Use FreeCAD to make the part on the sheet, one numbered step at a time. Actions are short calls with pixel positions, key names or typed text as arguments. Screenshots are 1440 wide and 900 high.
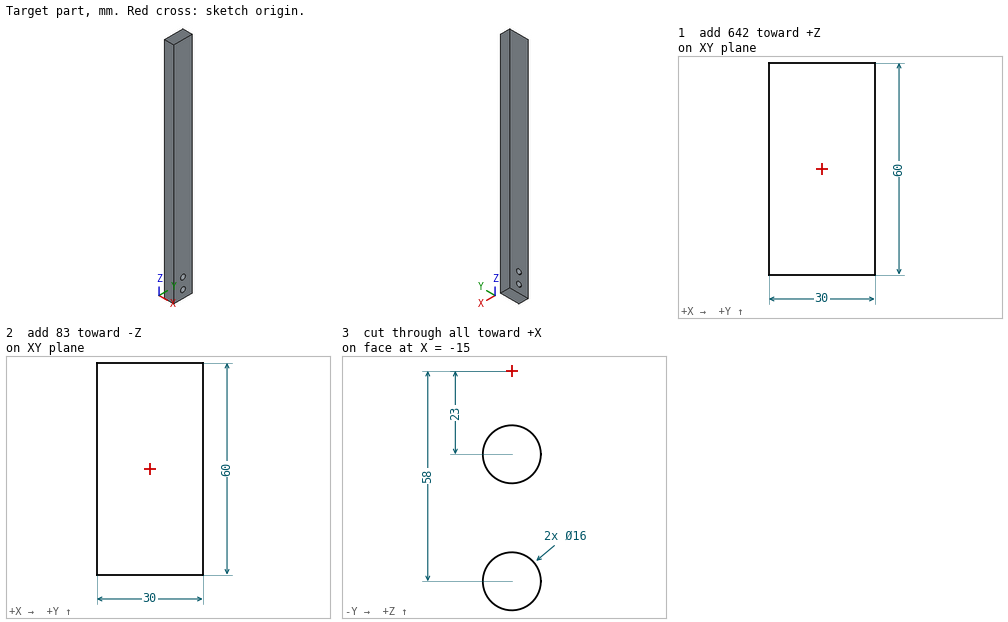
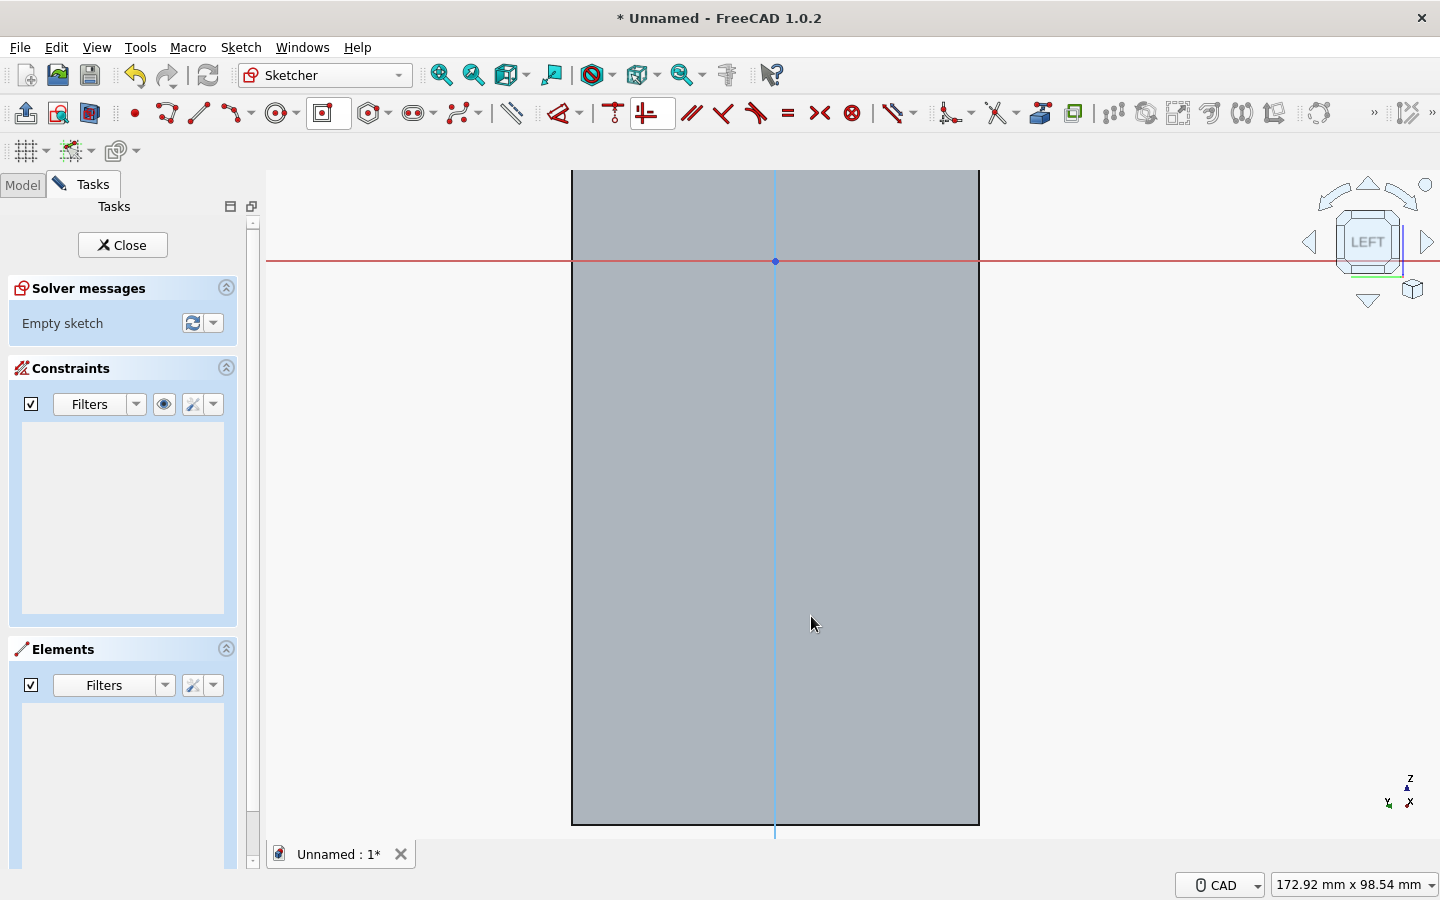
click(276, 114)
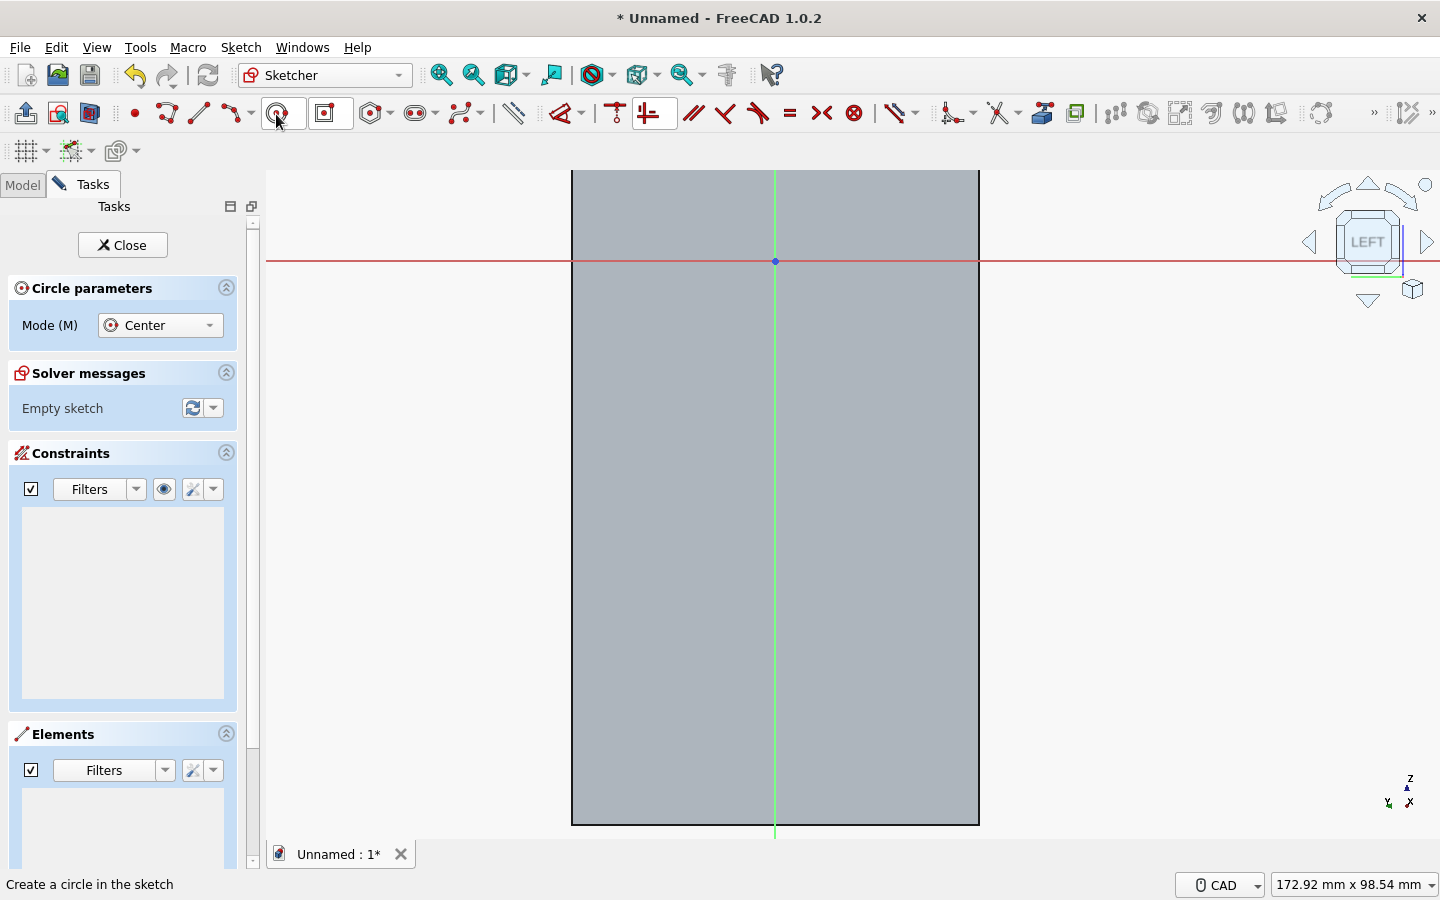
click(775, 655)
move(814, 617)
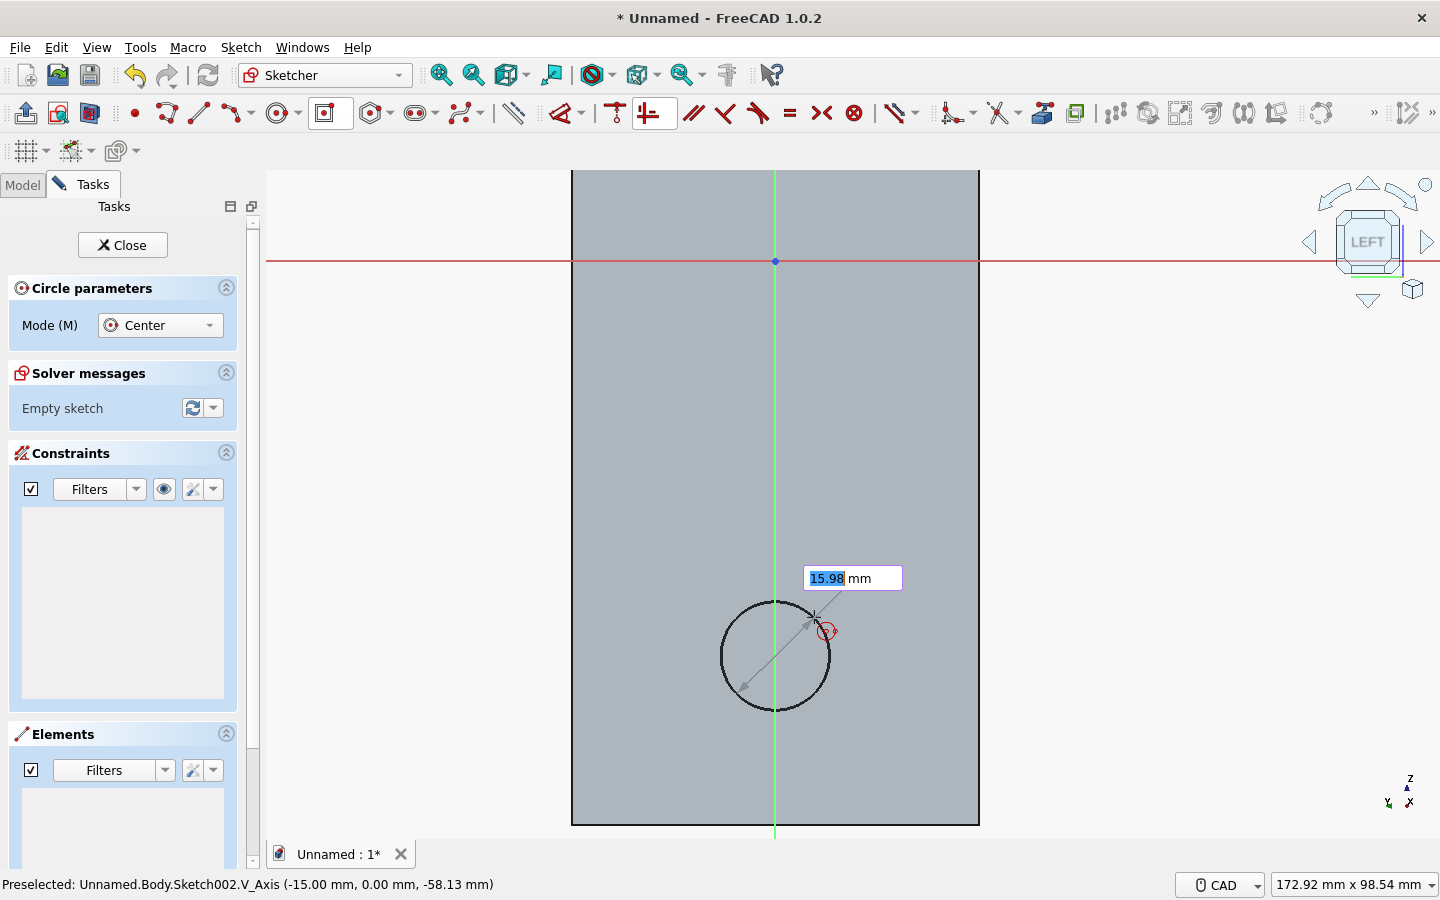
text(16)
key(Return)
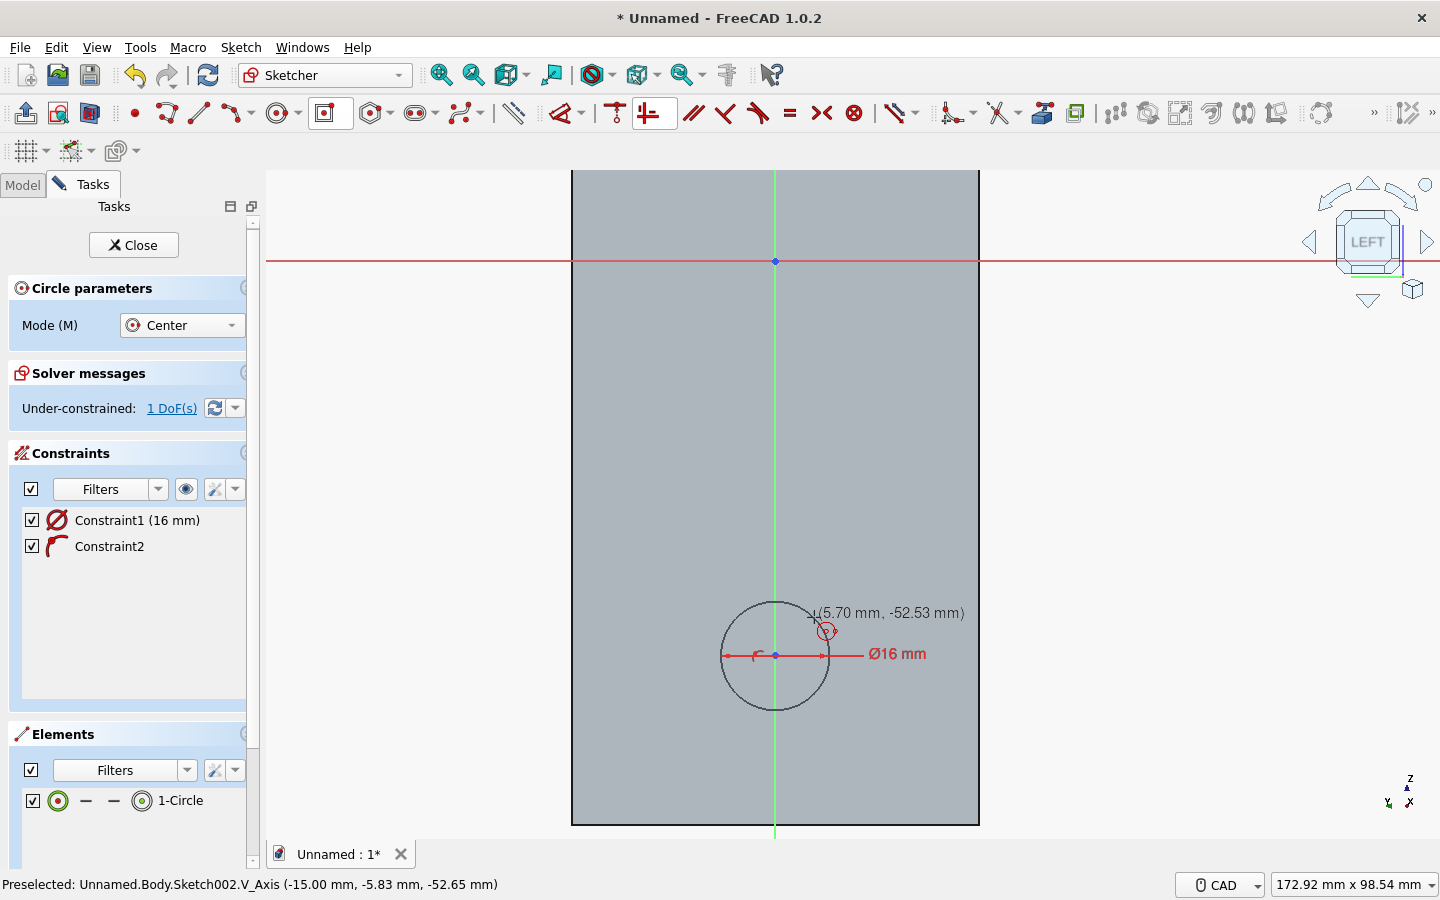
click(775, 417)
move(814, 379)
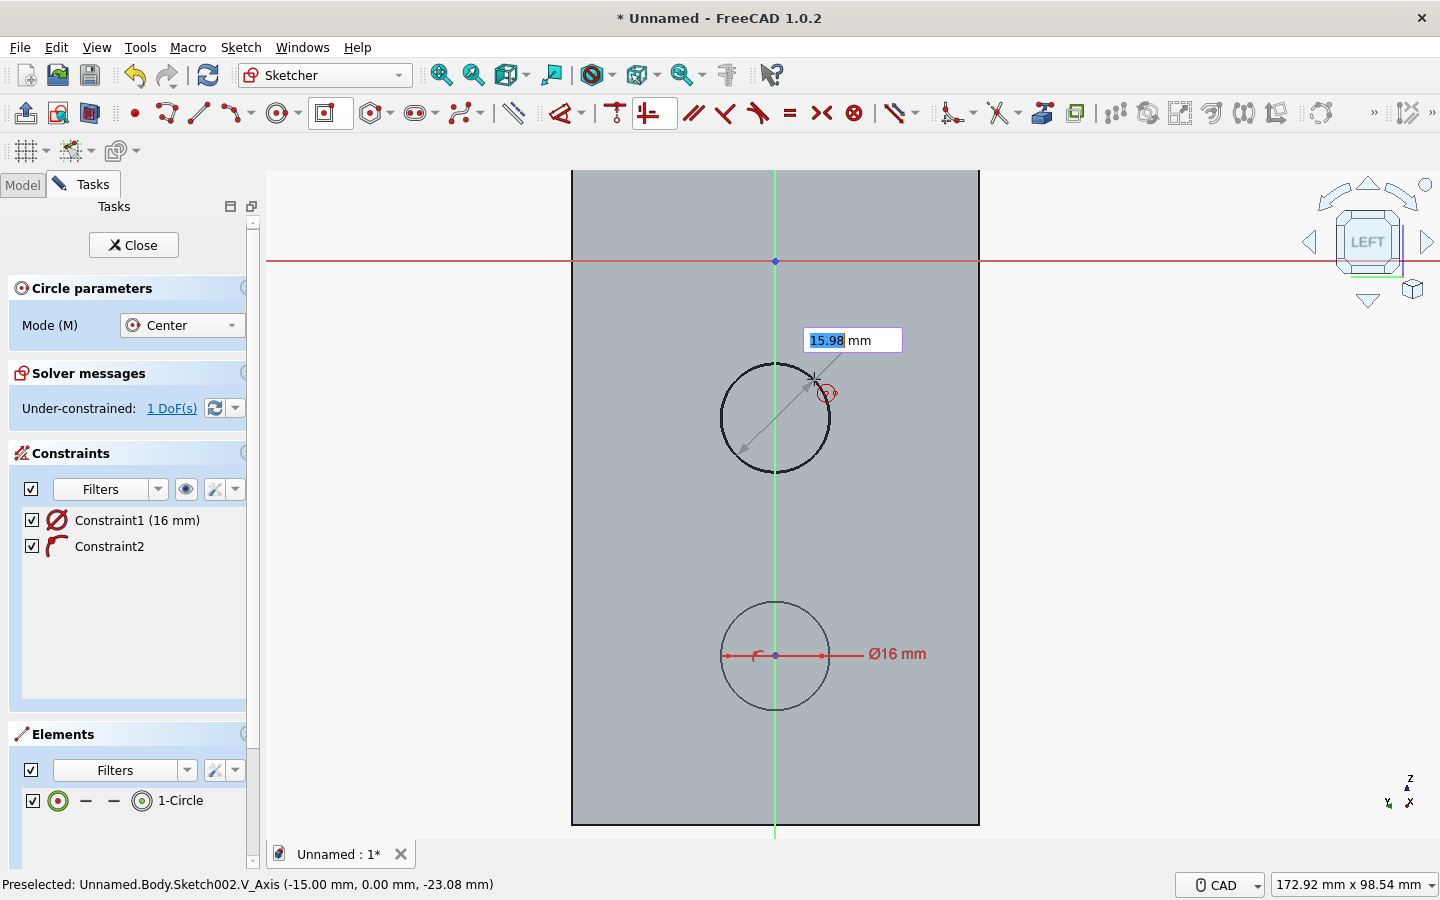
text(16)
key(Return)
key(Escape)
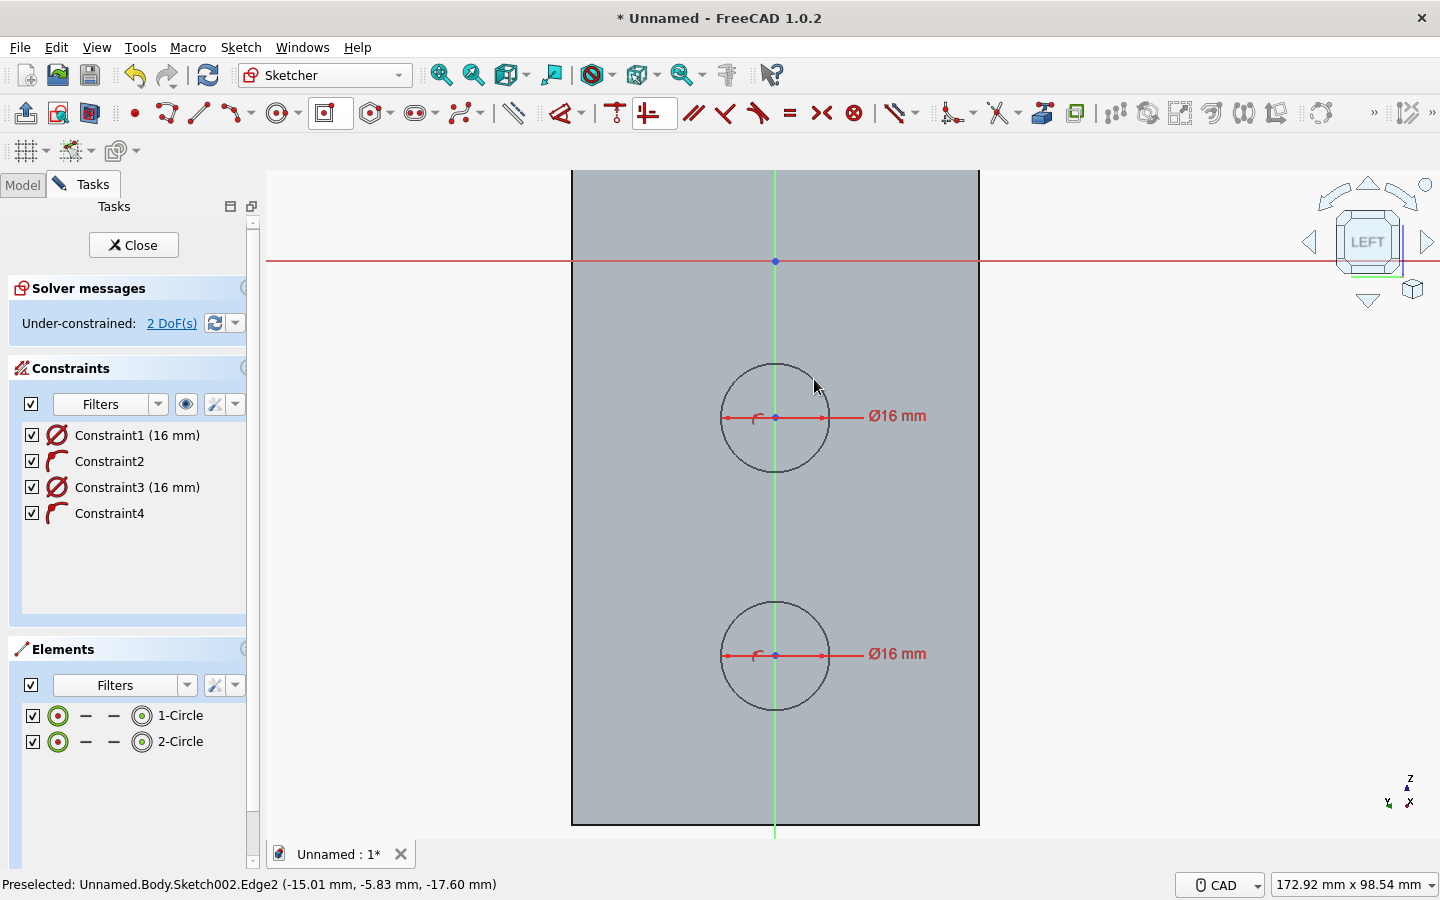
click(775, 656)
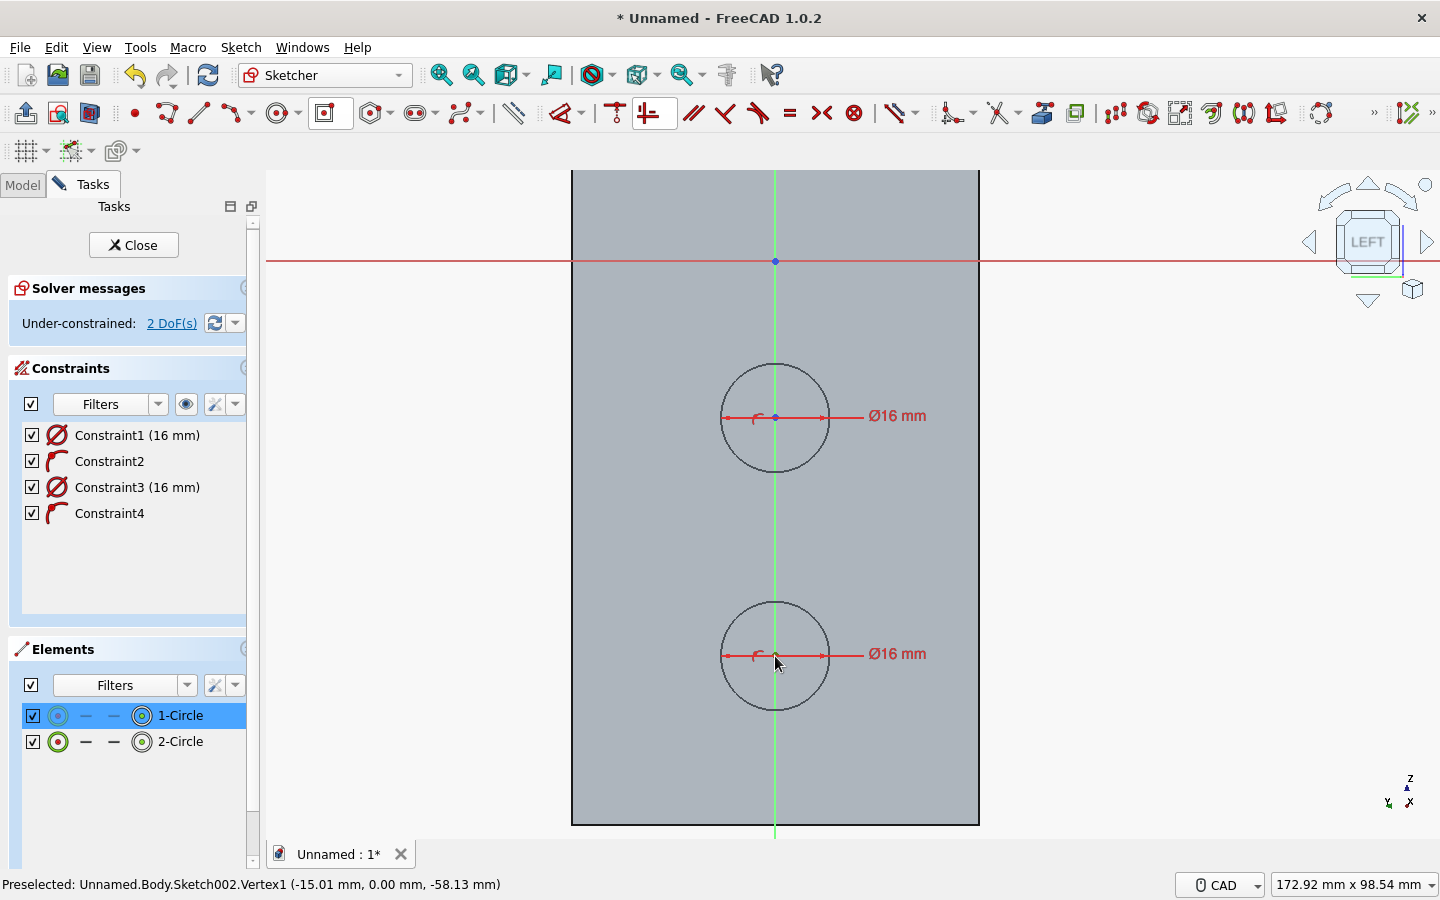
key(i)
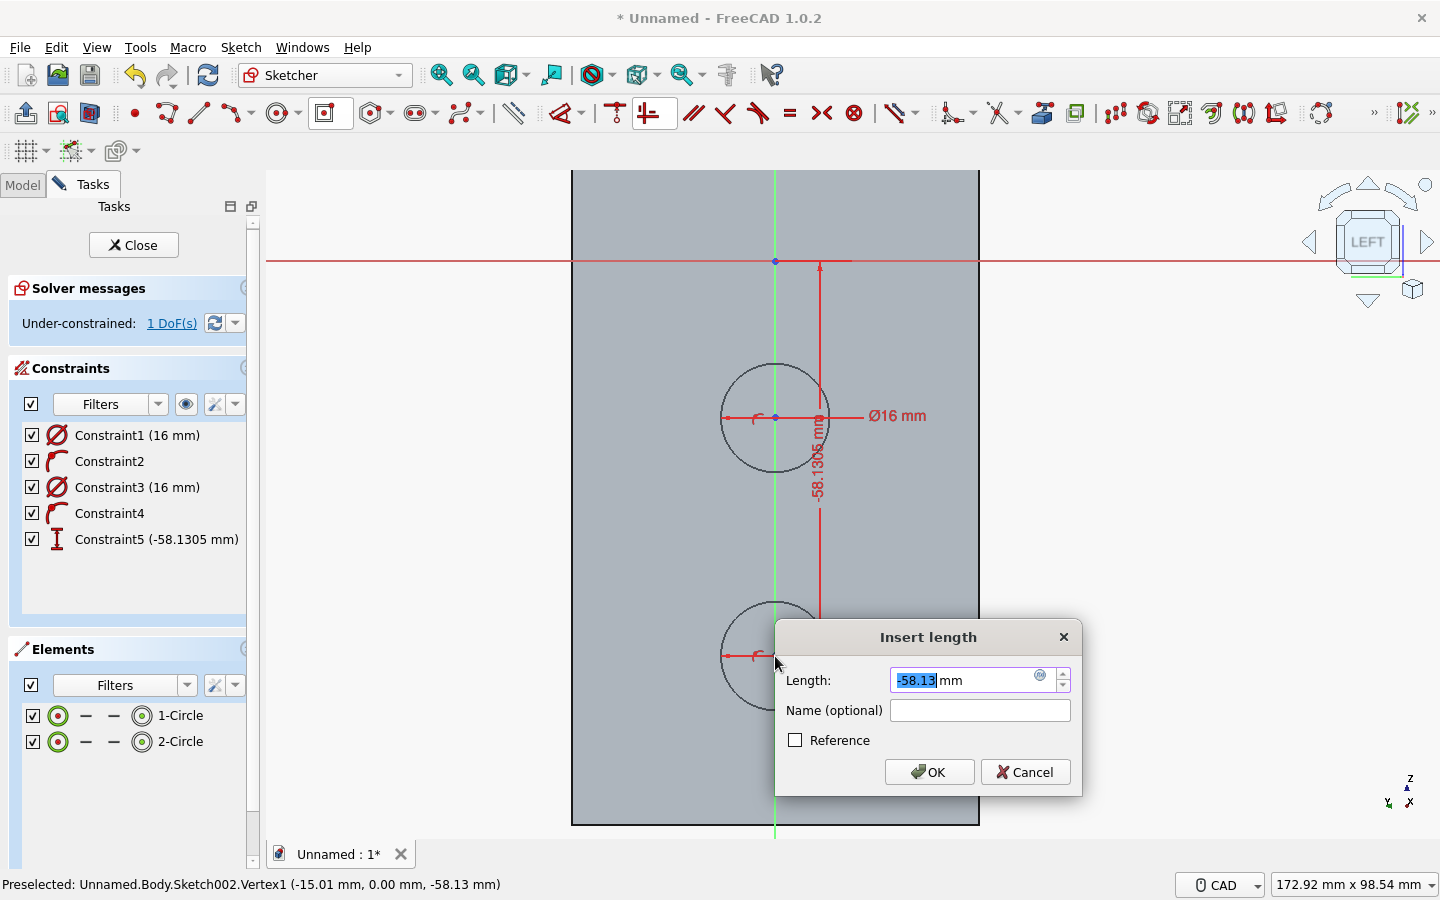
text(-58)
key(Return)